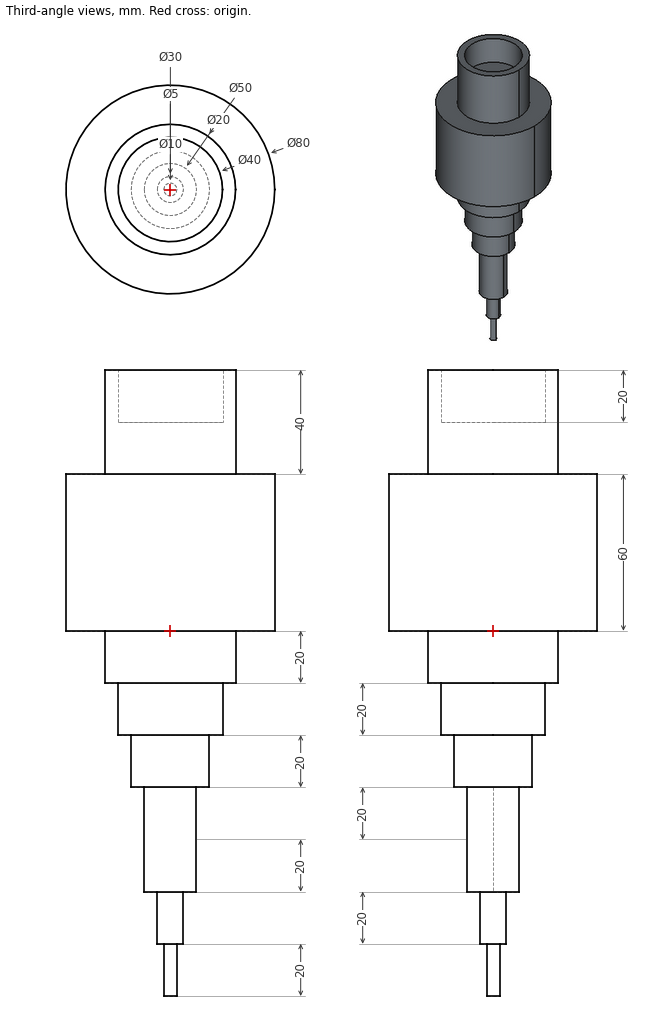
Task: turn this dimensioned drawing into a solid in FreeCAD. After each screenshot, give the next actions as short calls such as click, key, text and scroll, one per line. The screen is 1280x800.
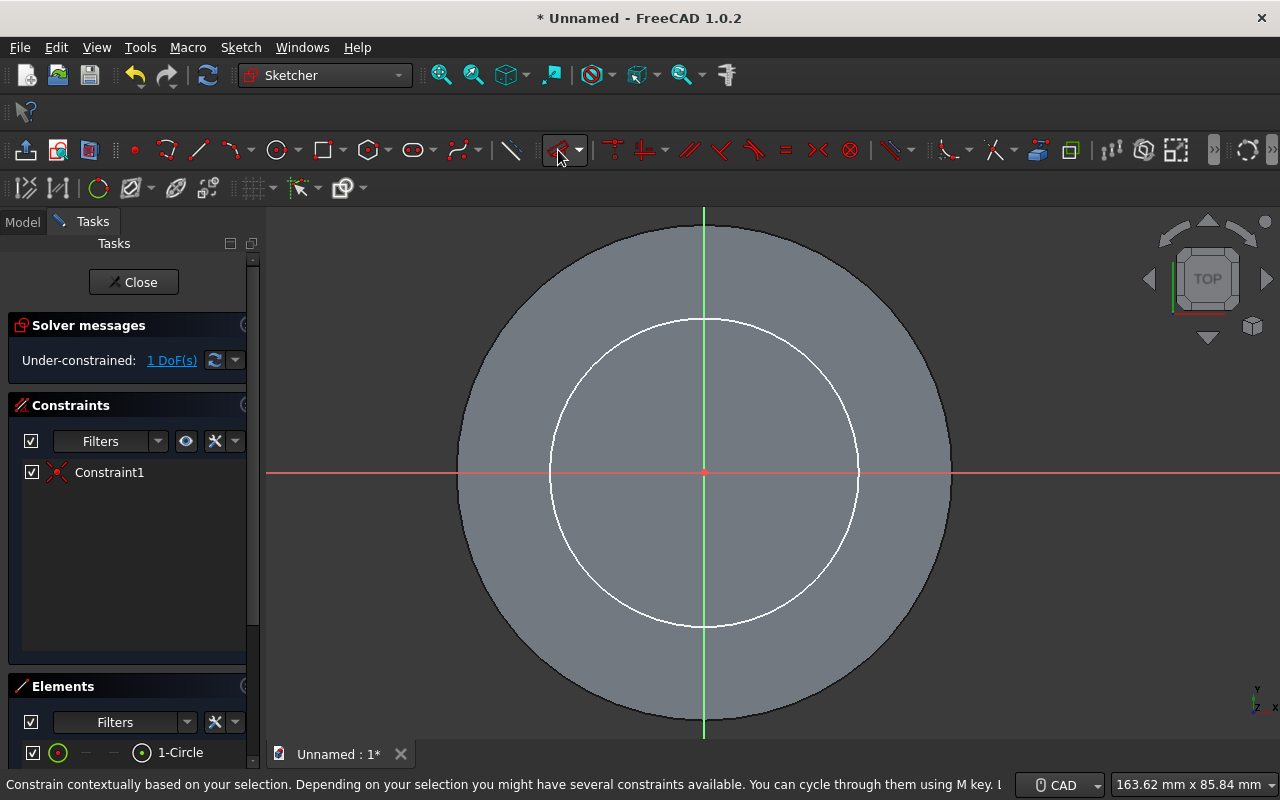
click(813, 363)
click(836, 340)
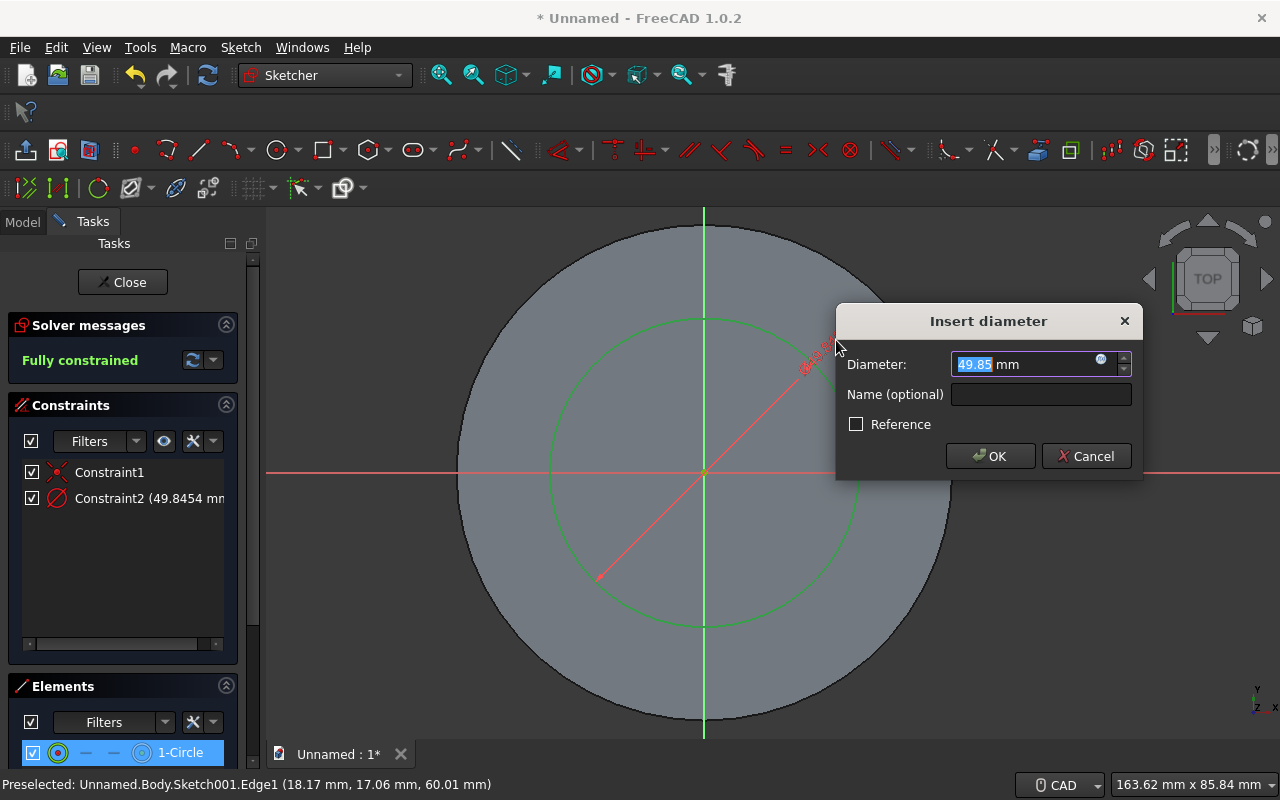
text(50)
key(Return)
key(Escape)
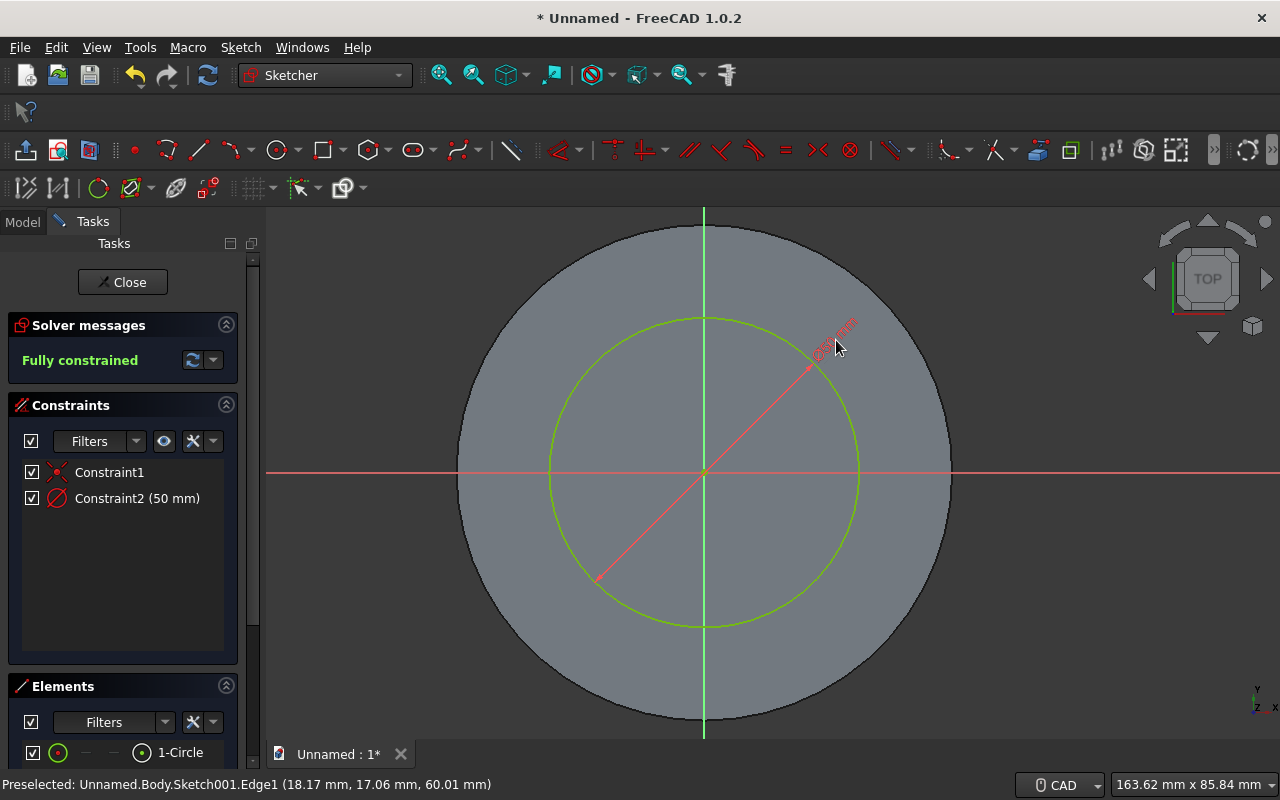
click(123, 282)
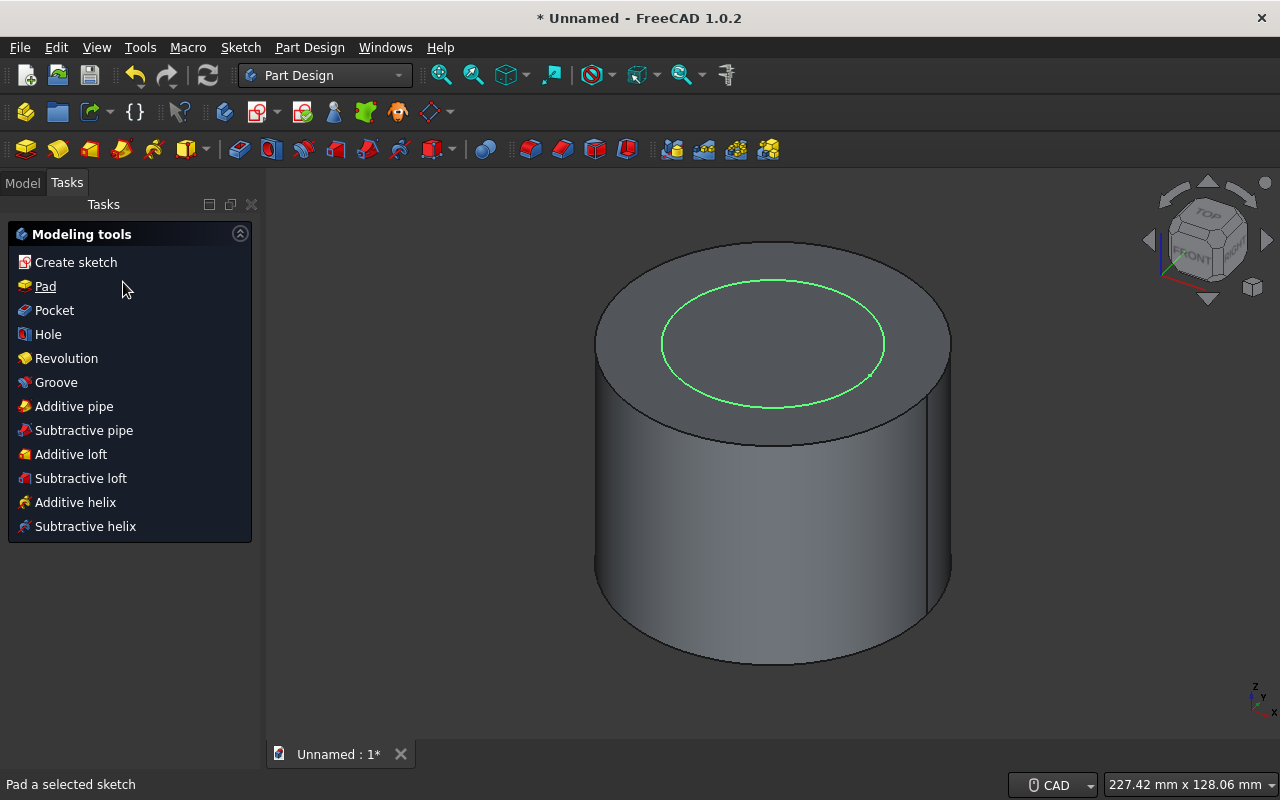
click(26, 150)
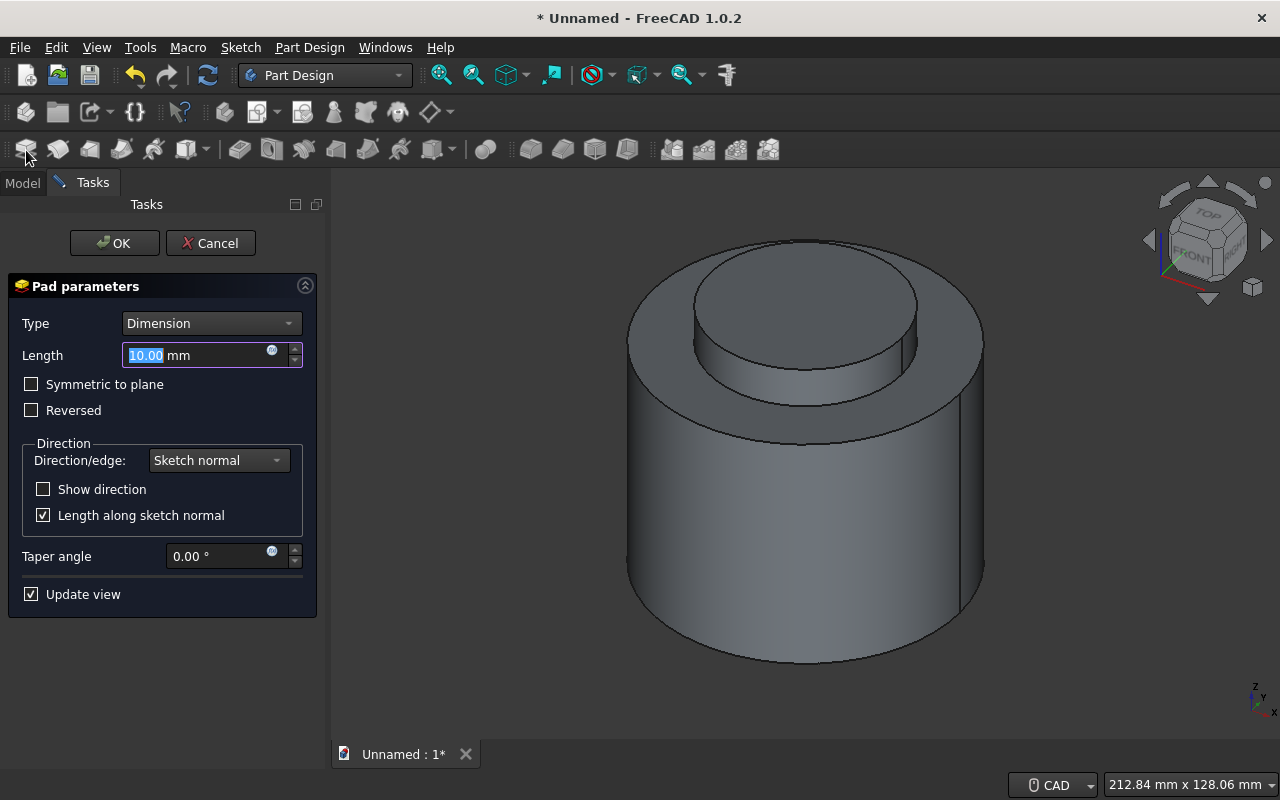
text(40)
key(Tab)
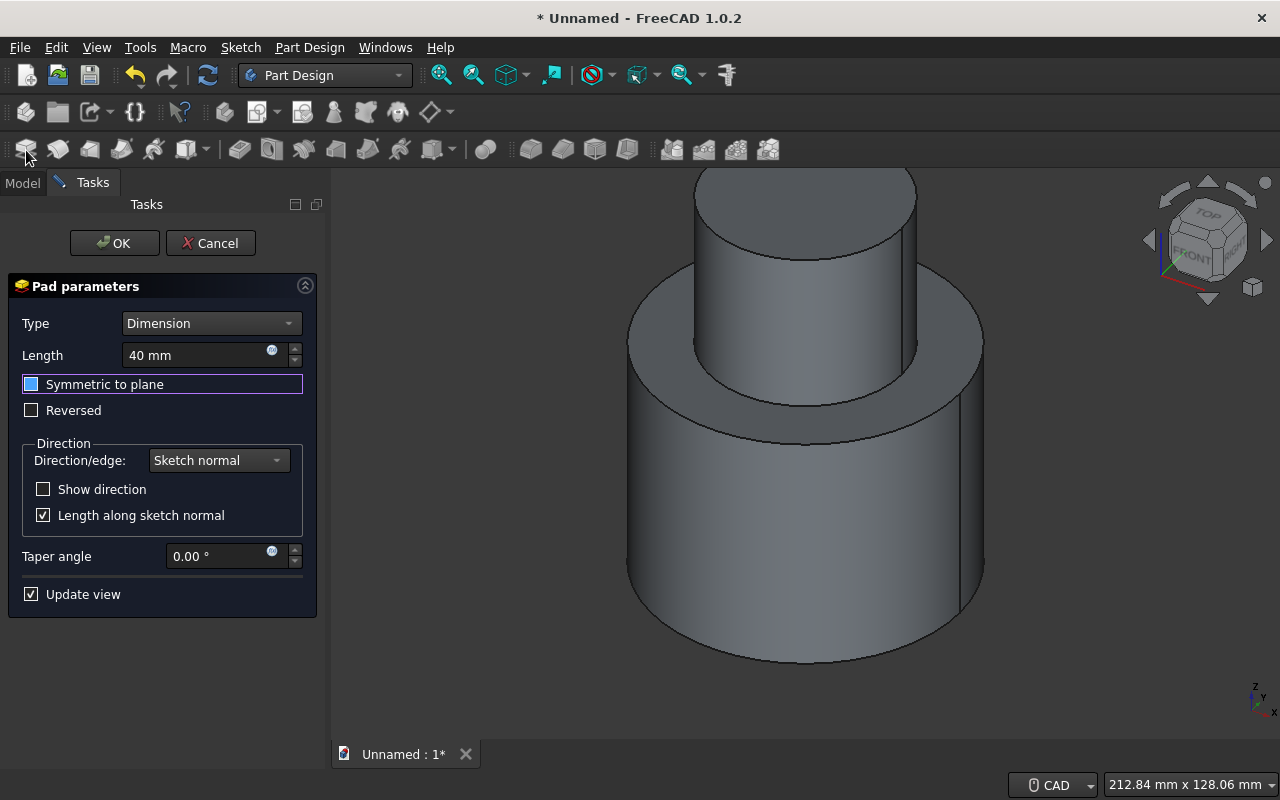
click(115, 243)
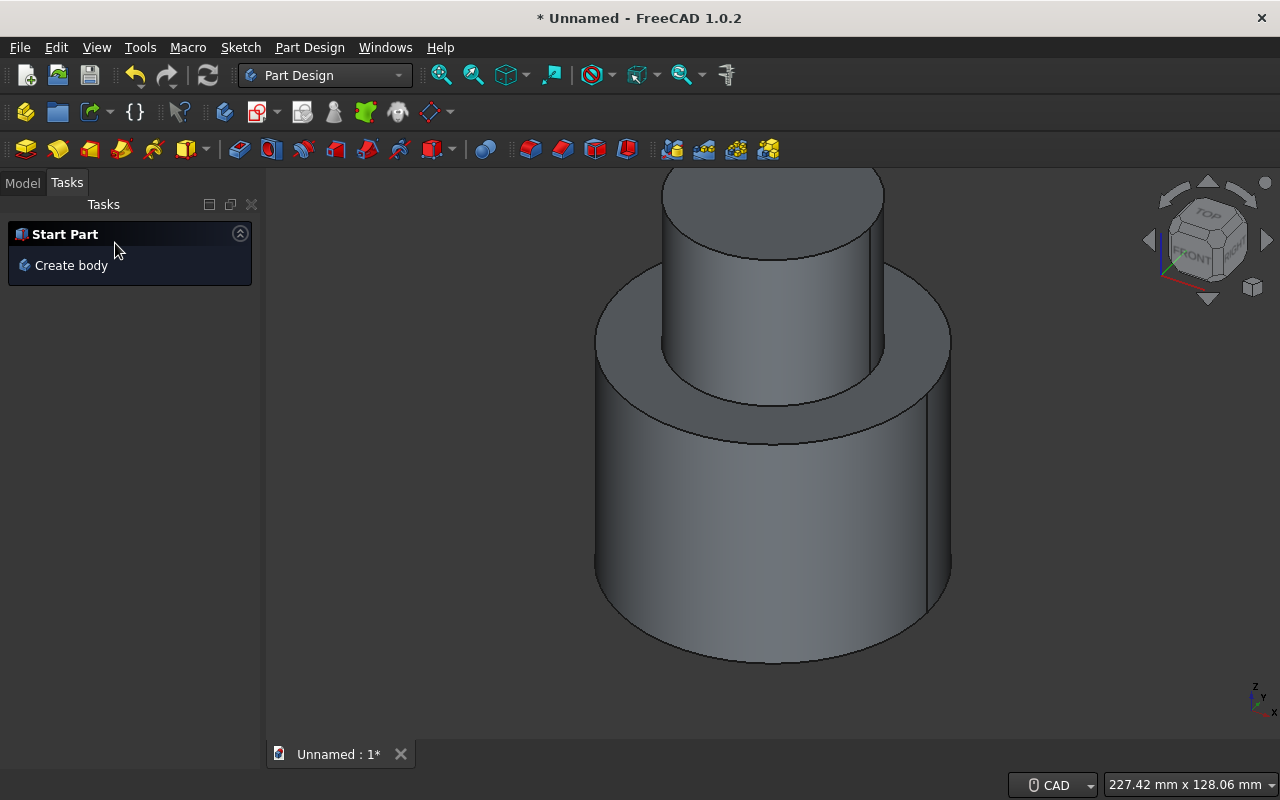
click(442, 76)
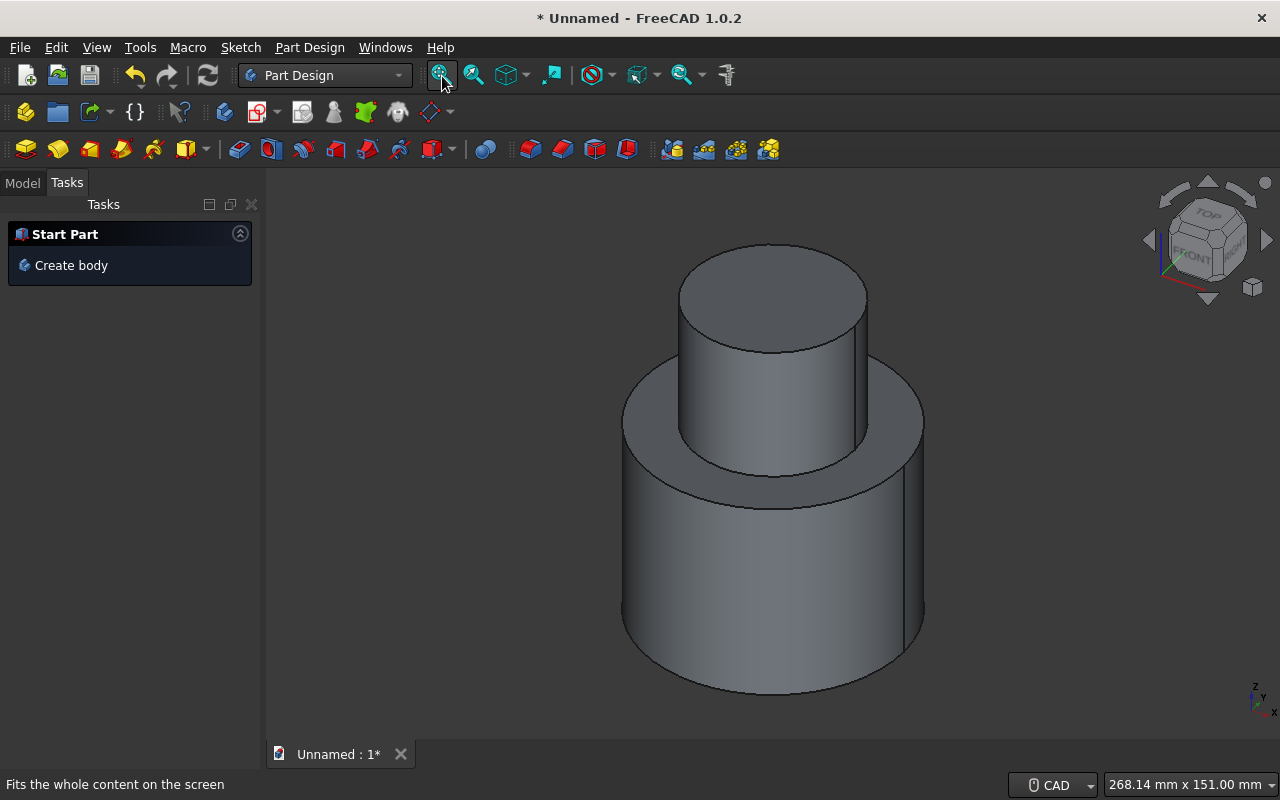
click(773, 298)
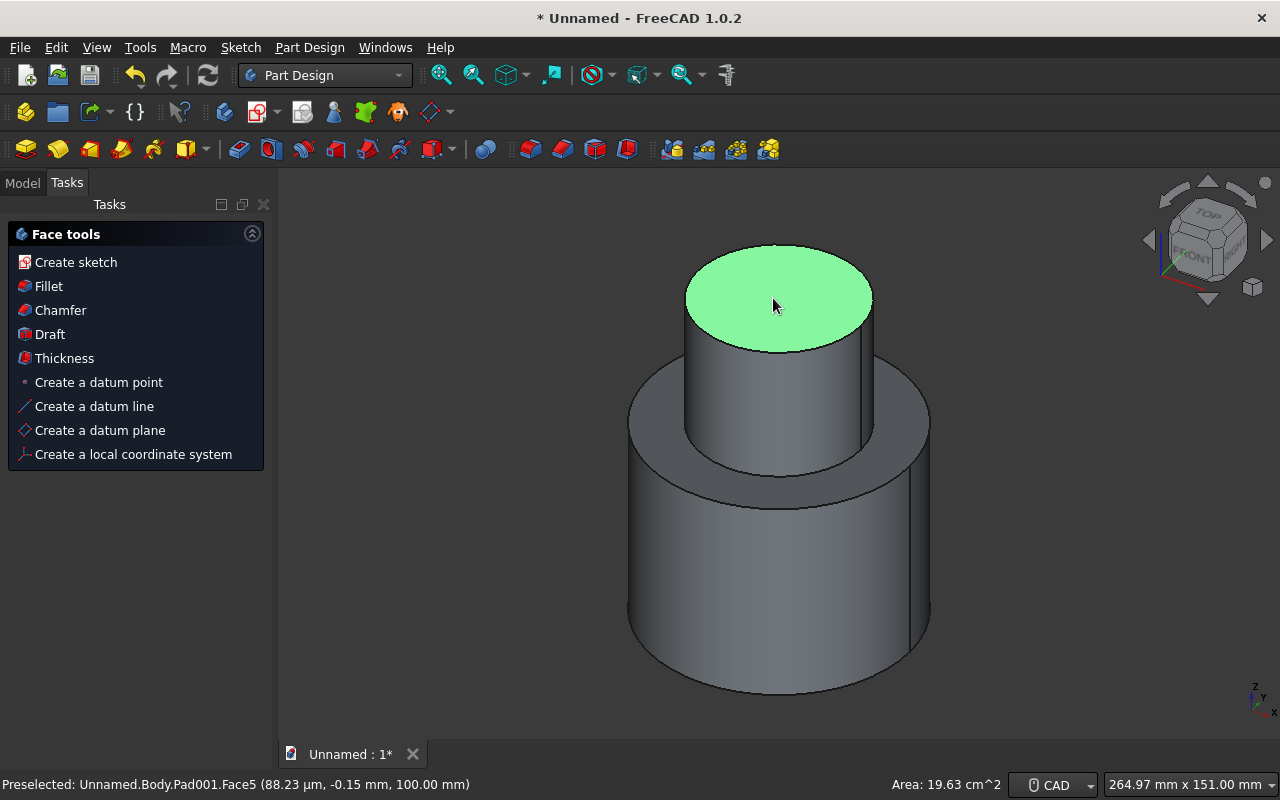
click(258, 112)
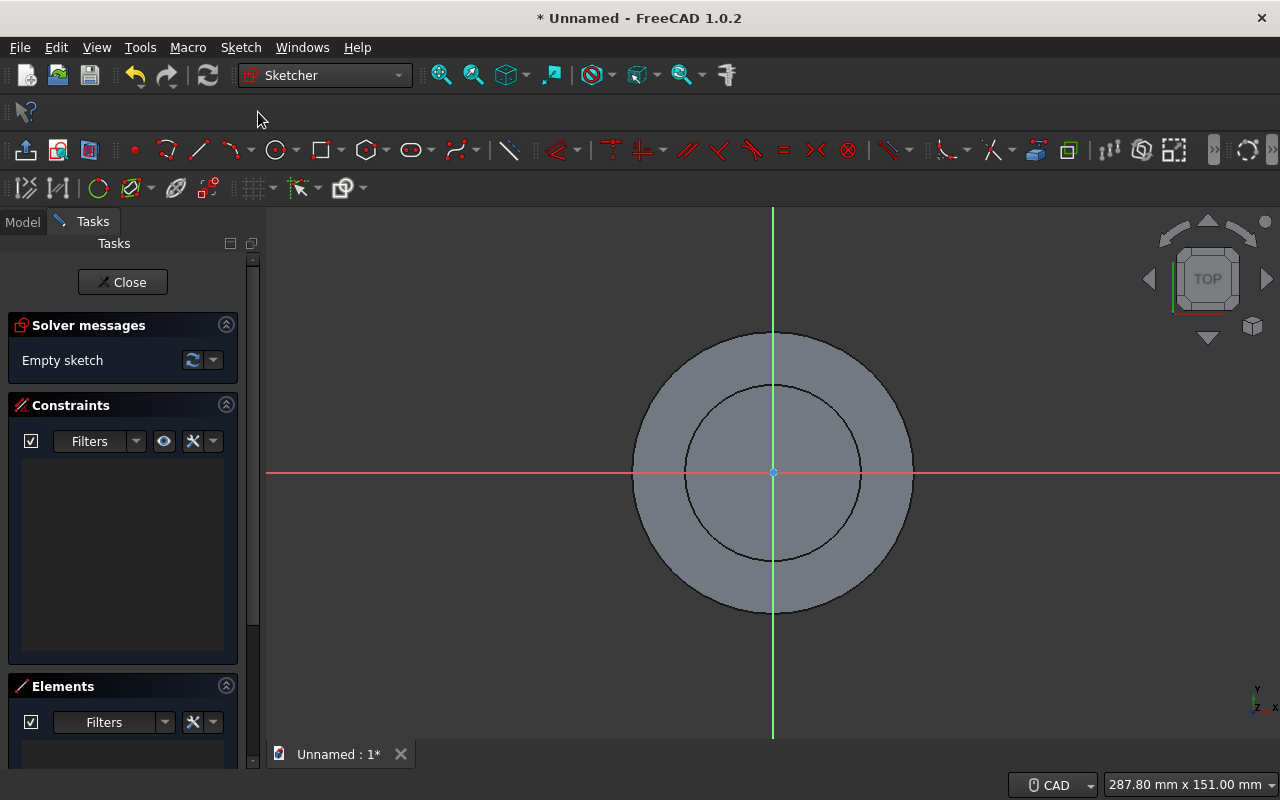
scroll(829, 473, up, 4)